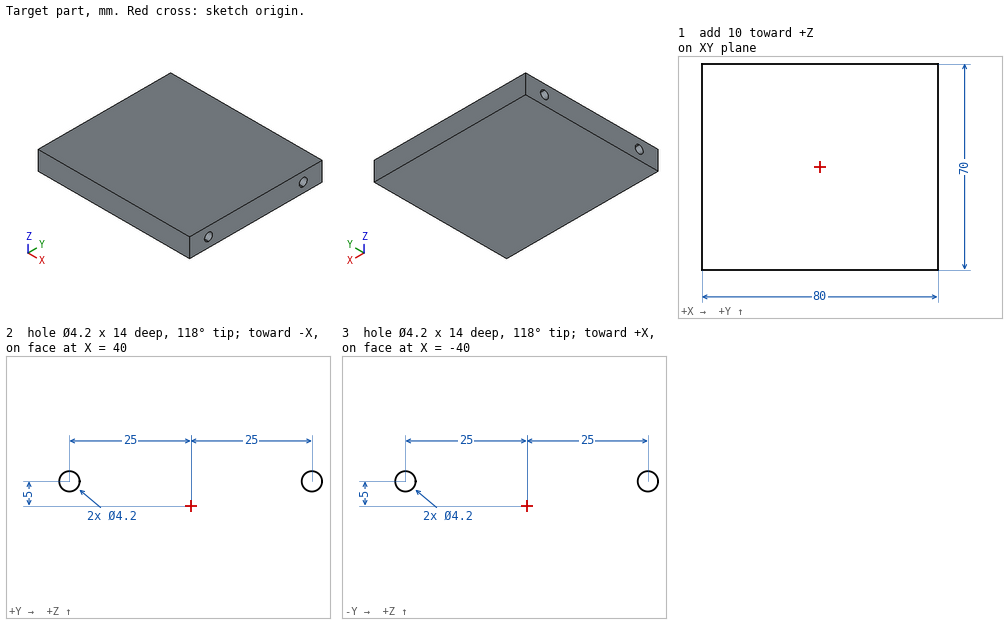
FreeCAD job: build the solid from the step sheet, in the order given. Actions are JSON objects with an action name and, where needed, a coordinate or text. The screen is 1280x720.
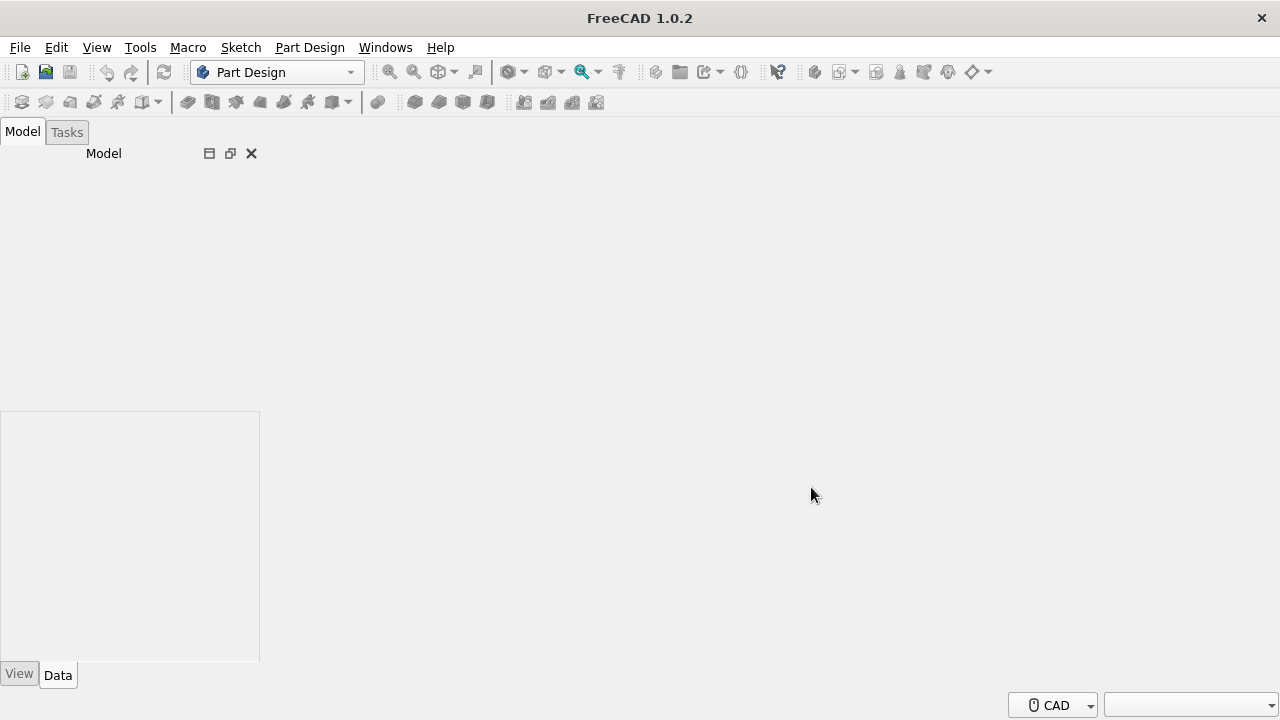
{"action": "left_click", "coordinate": [22, 72]}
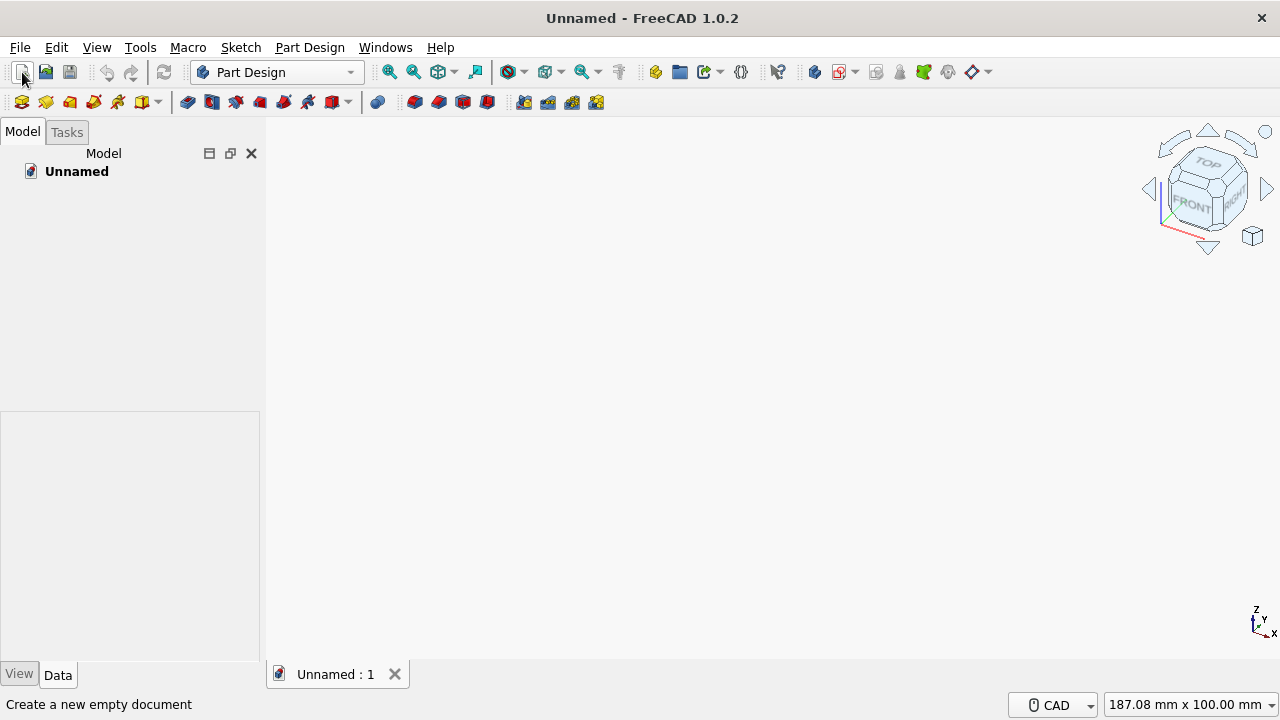
{"action": "left_click", "coordinate": [840, 72]}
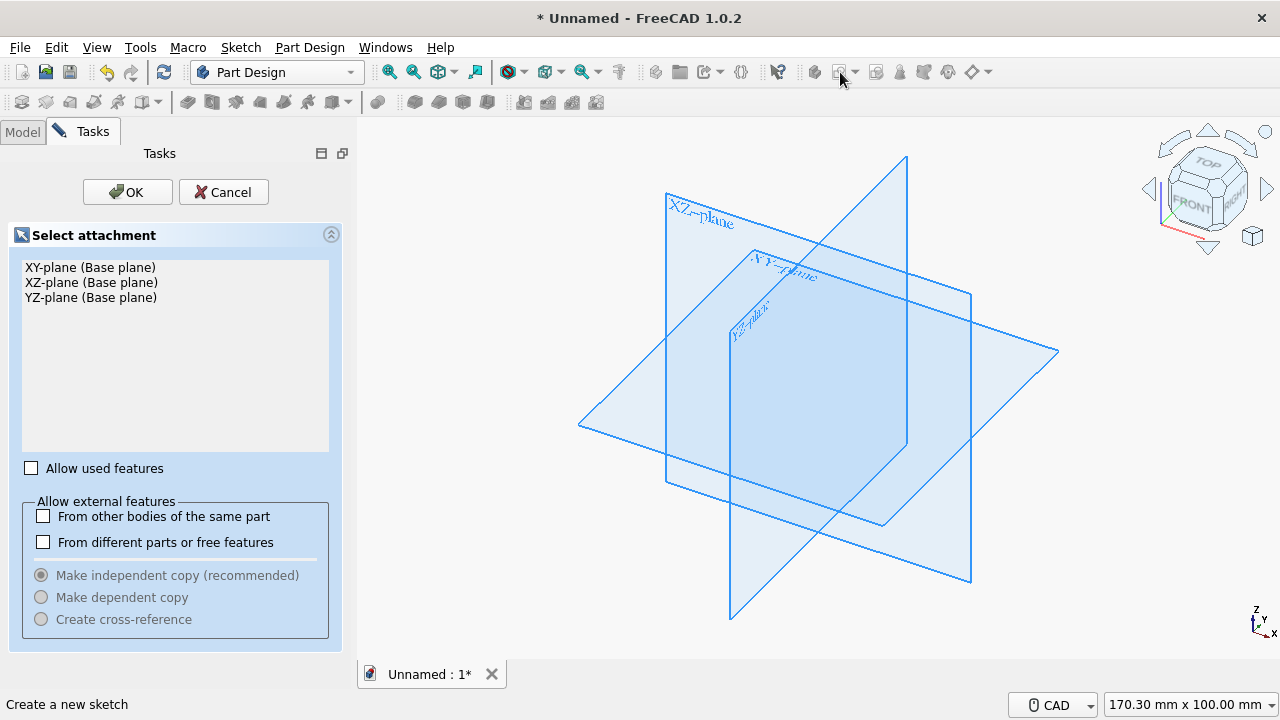
{"action": "left_click", "coordinate": [82, 268]}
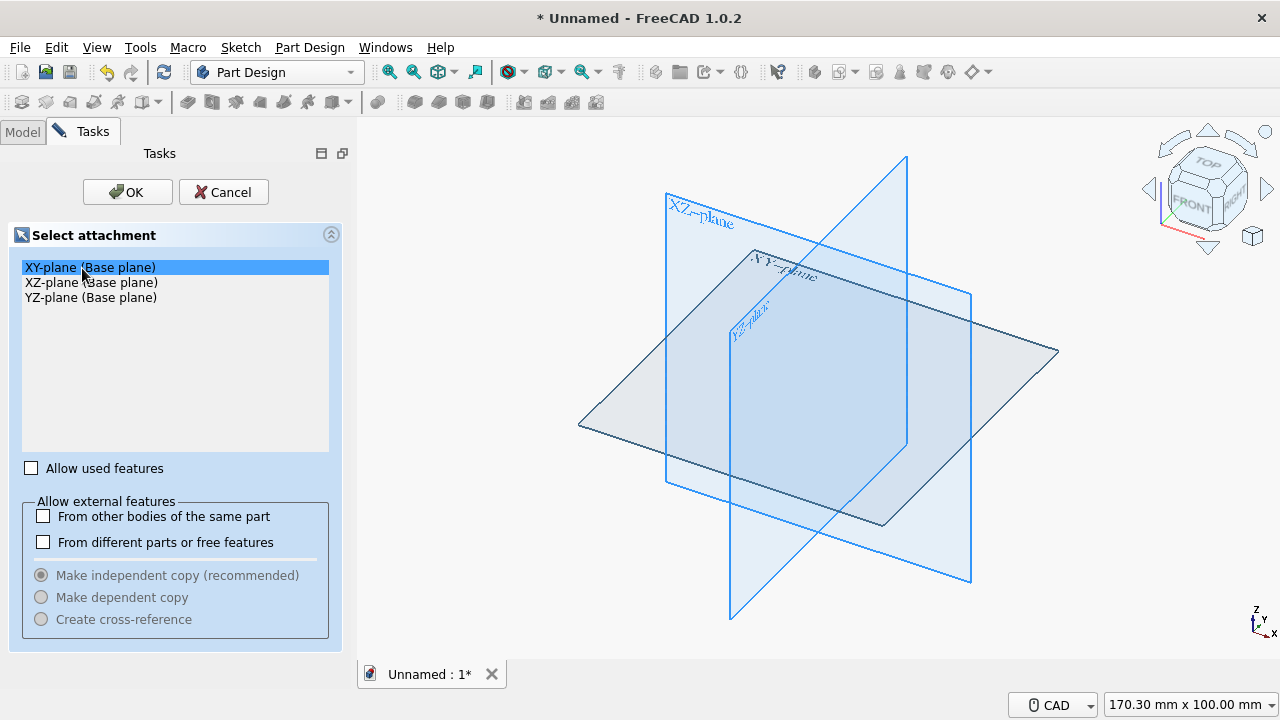
{"action": "left_click", "coordinate": [128, 192]}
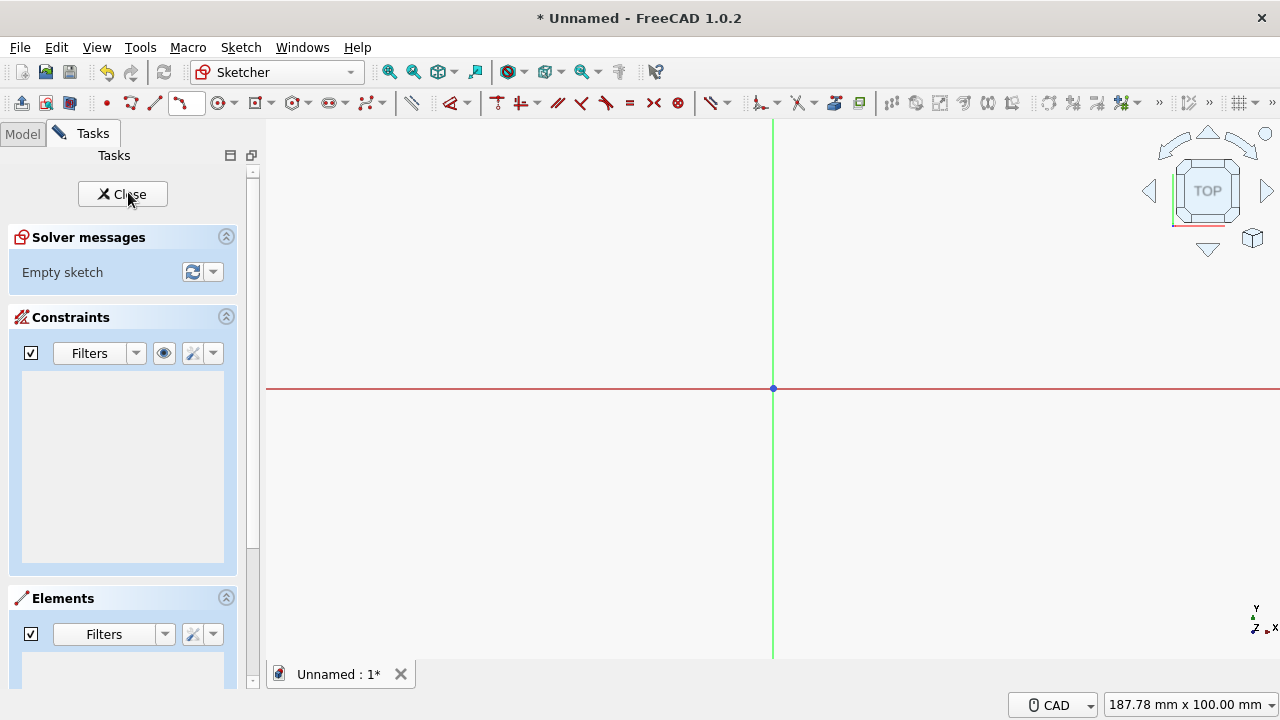
{"action": "left_click", "coordinate": [256, 104]}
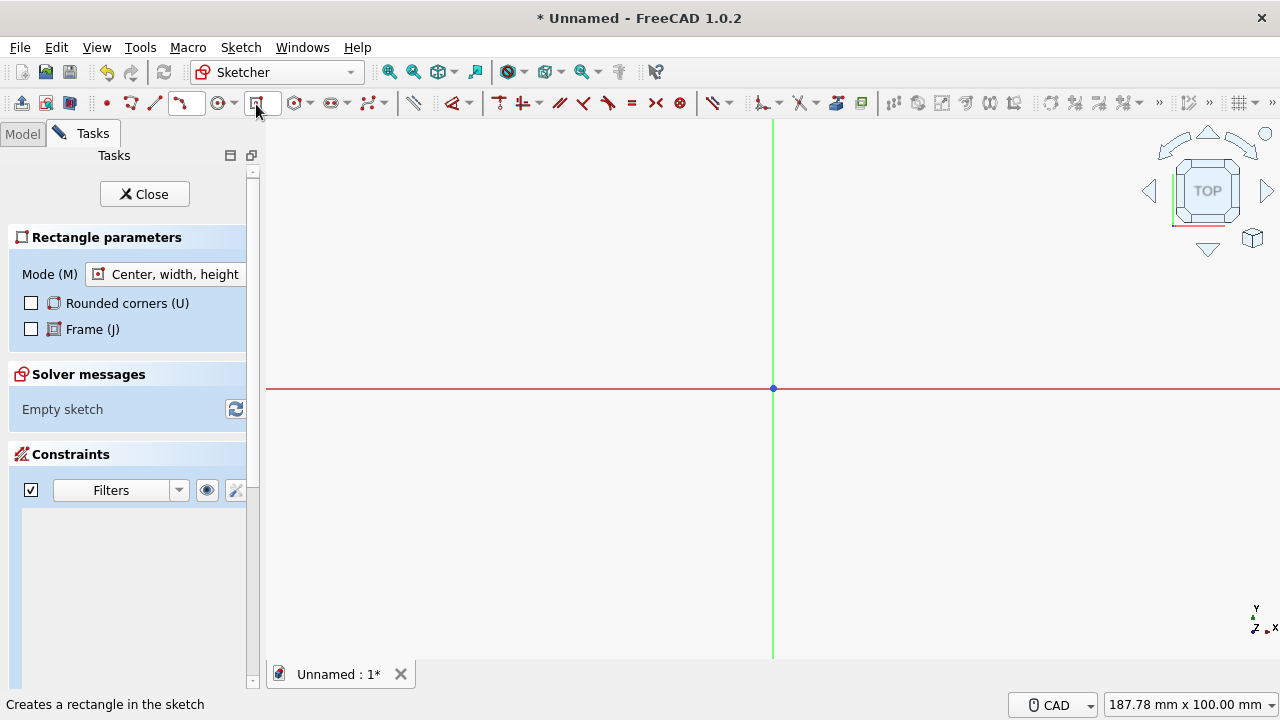
{"action": "left_click", "coordinate": [773, 389]}
{"action": "left_click", "coordinate": [989, 200]}
{"action": "key", "text": "Escape"}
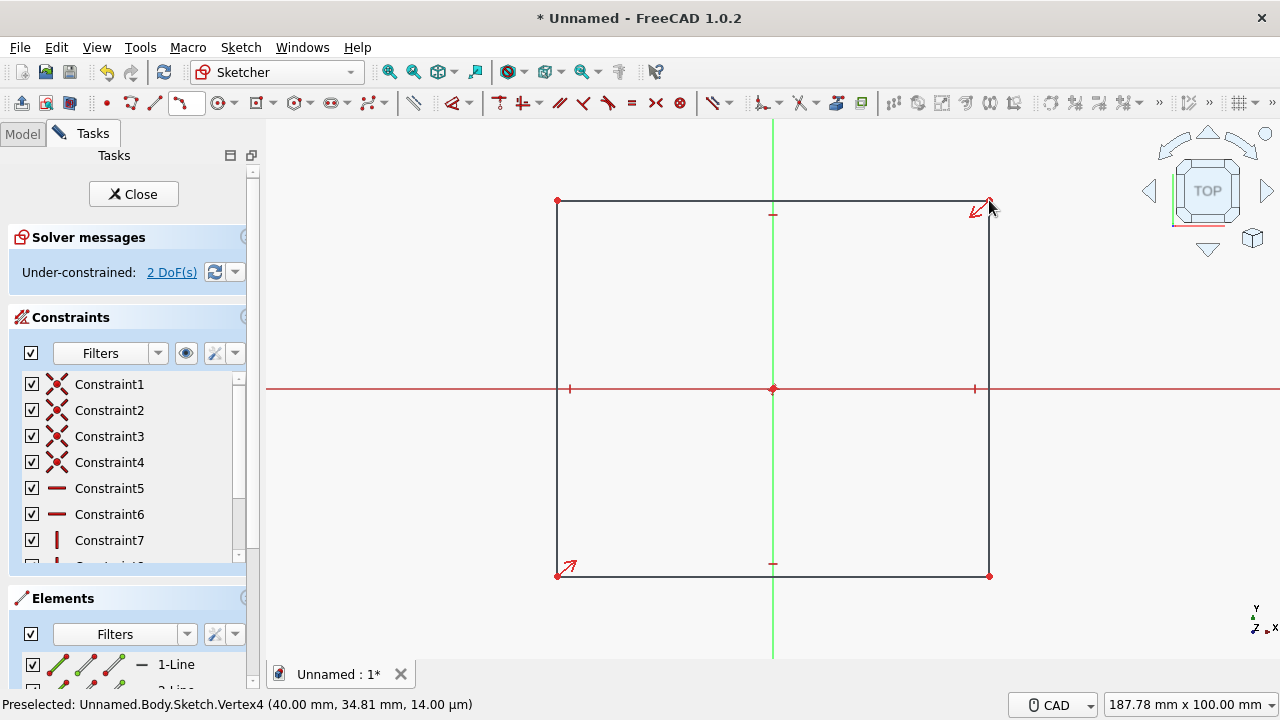
{"action": "key", "text": "d"}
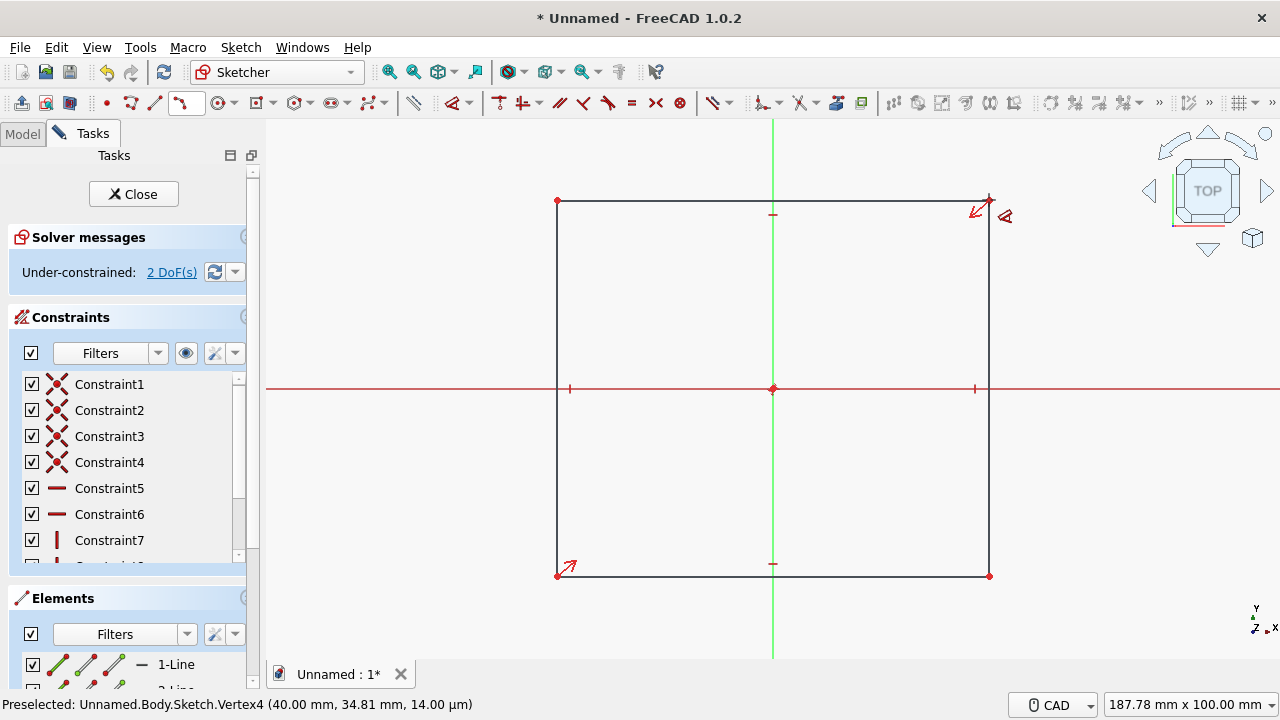
{"action": "left_click", "coordinate": [687, 577]}
{"action": "left_click", "coordinate": [674, 611]}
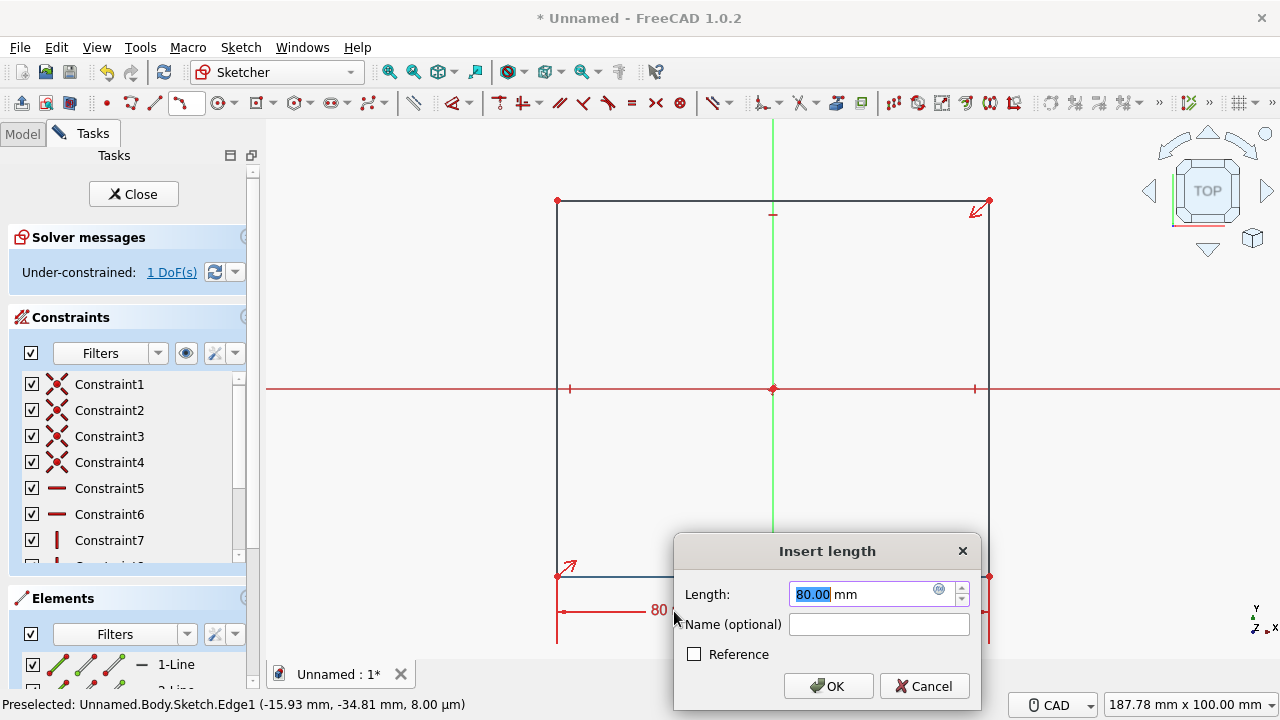
{"action": "type", "text": "80"}
{"action": "key", "text": "Return"}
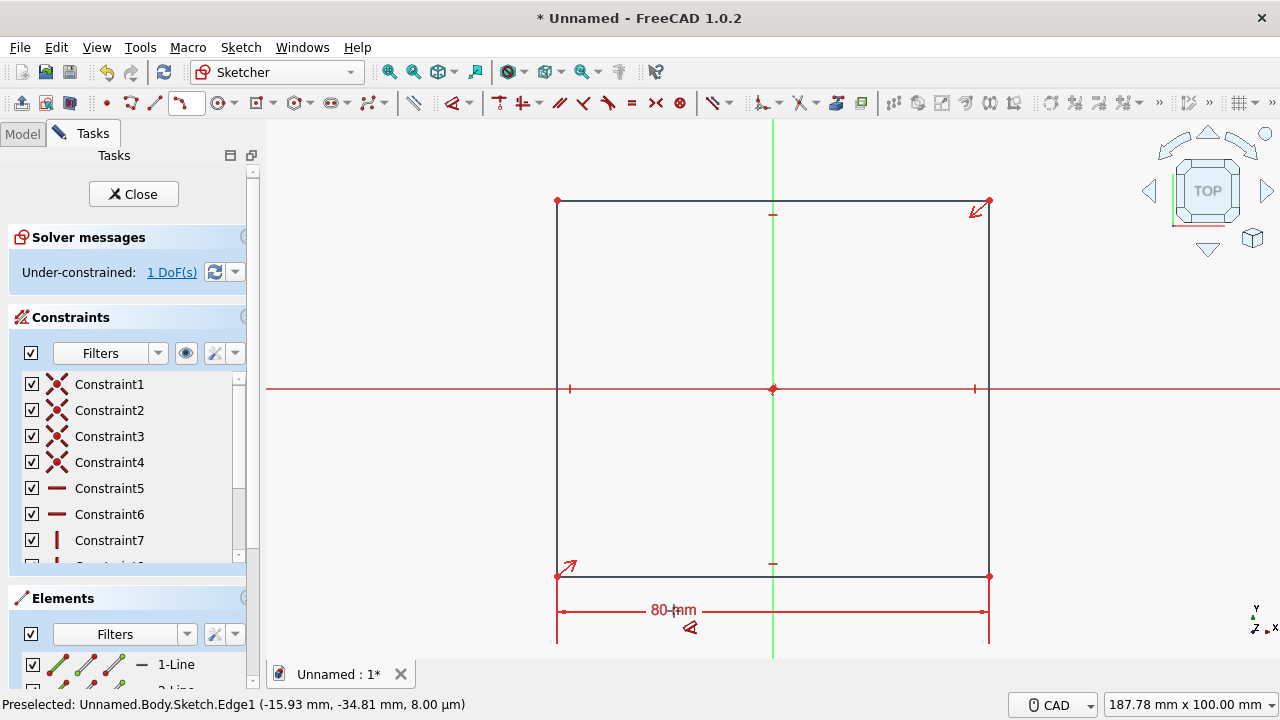
{"action": "left_click", "coordinate": [989, 464]}
{"action": "left_click", "coordinate": [1023, 303]}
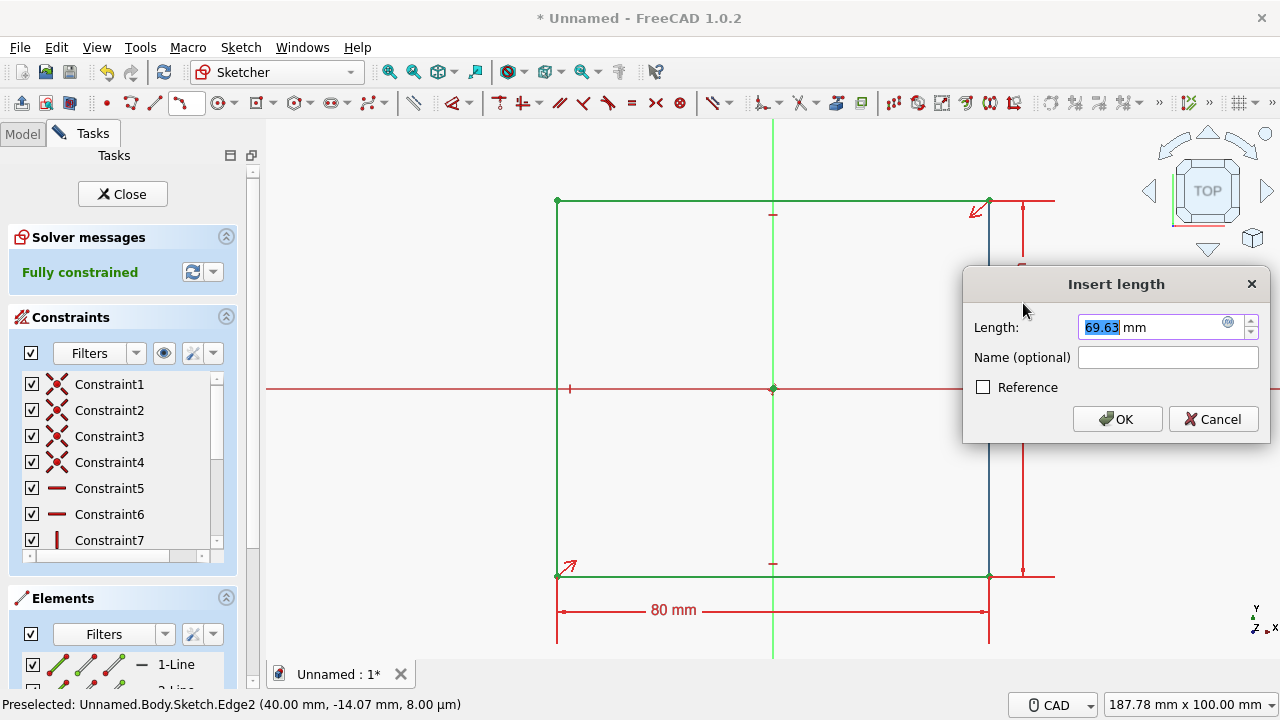
{"action": "type", "text": "70"}
{"action": "key", "text": "Return"}
{"action": "key", "text": "Escape"}